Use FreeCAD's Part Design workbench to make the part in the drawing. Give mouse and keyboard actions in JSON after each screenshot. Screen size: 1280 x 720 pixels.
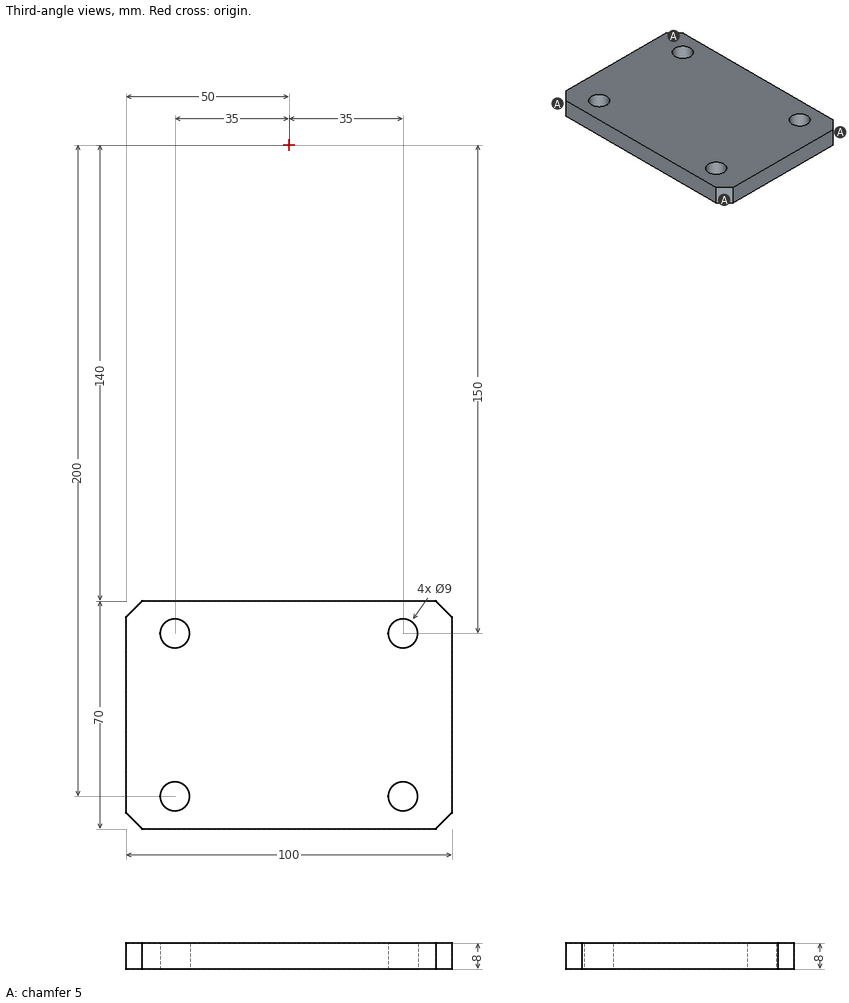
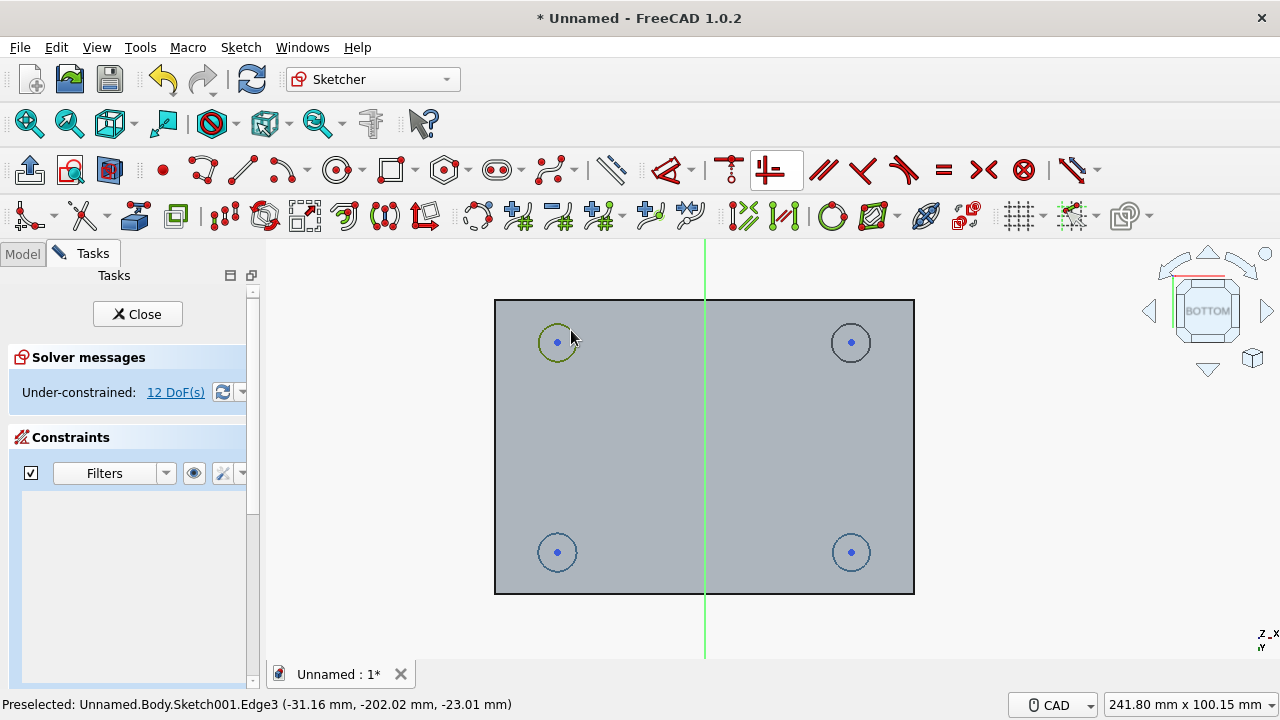
{"action": "left_click", "coordinate": [864, 329]}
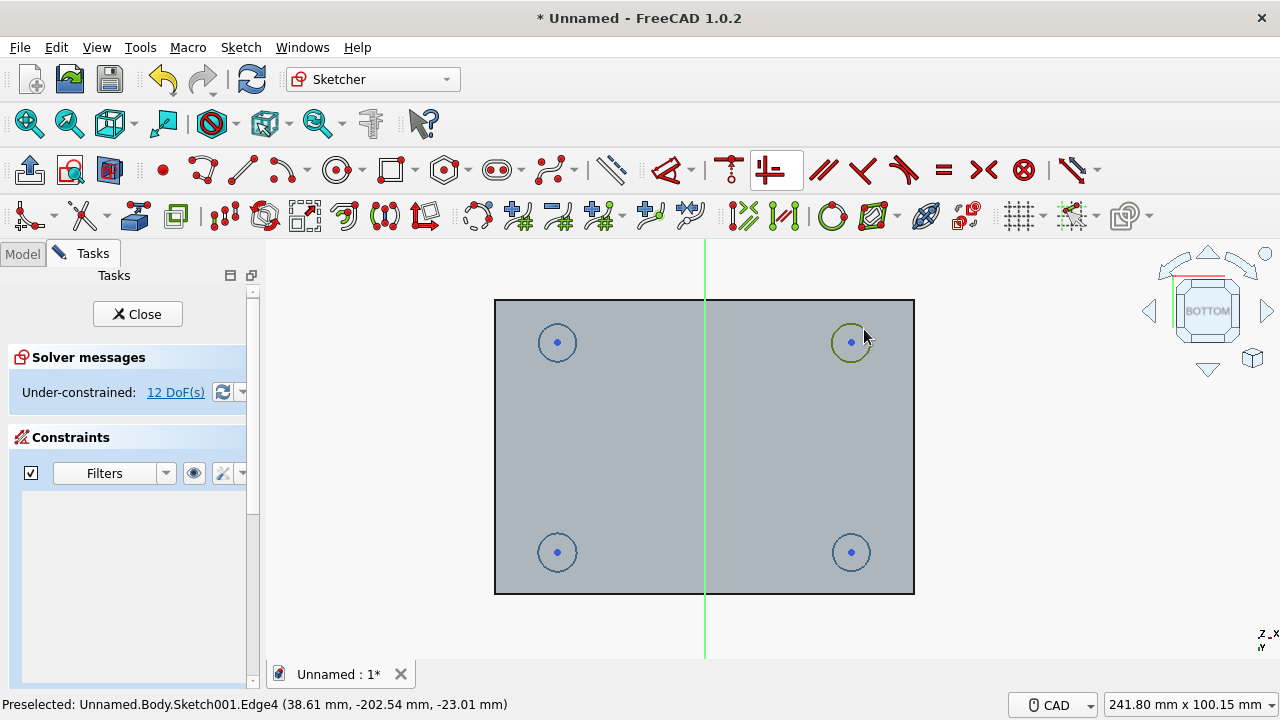
{"action": "left_click", "coordinate": [944, 170]}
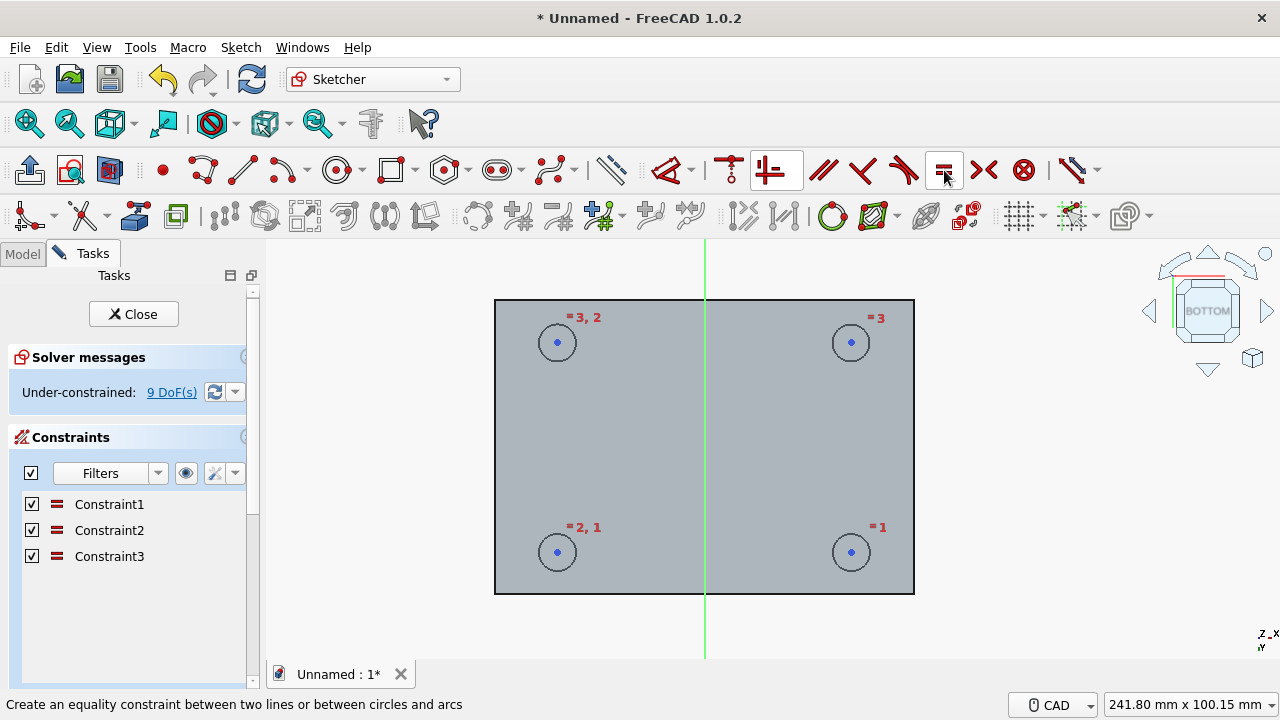
{"action": "left_click", "coordinate": [851, 553]}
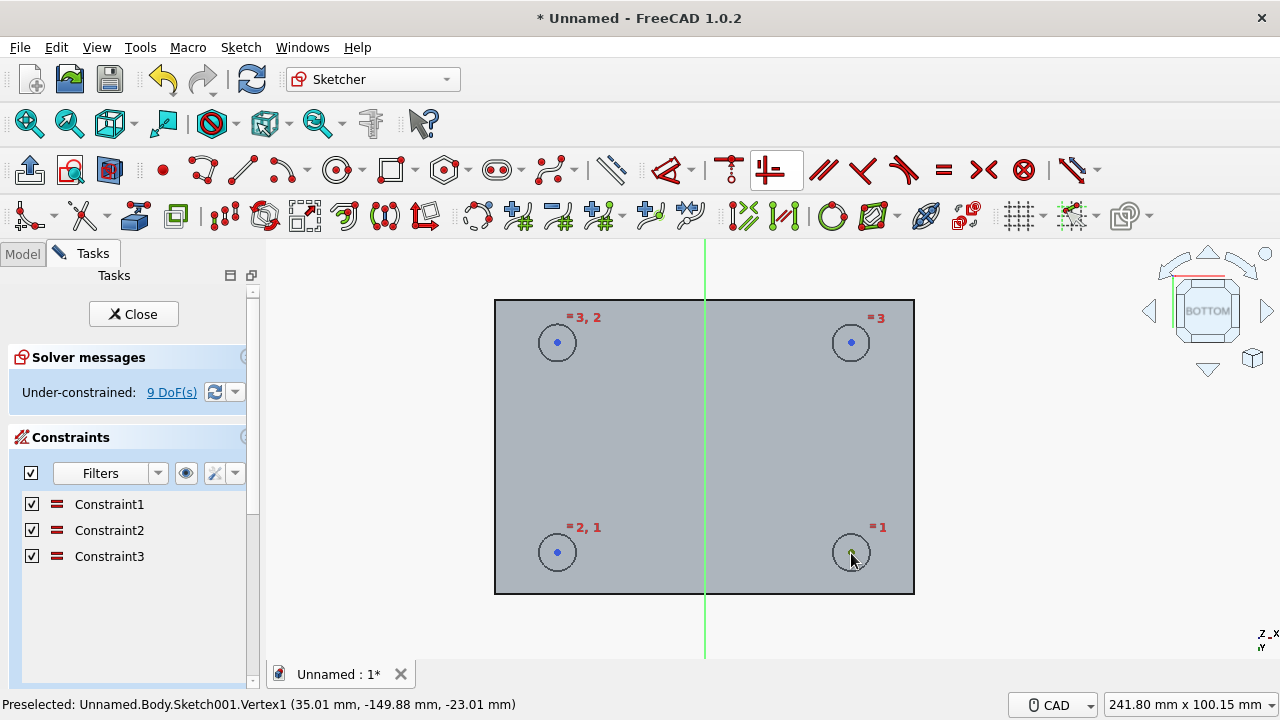
{"action": "left_click", "coordinate": [557, 553]}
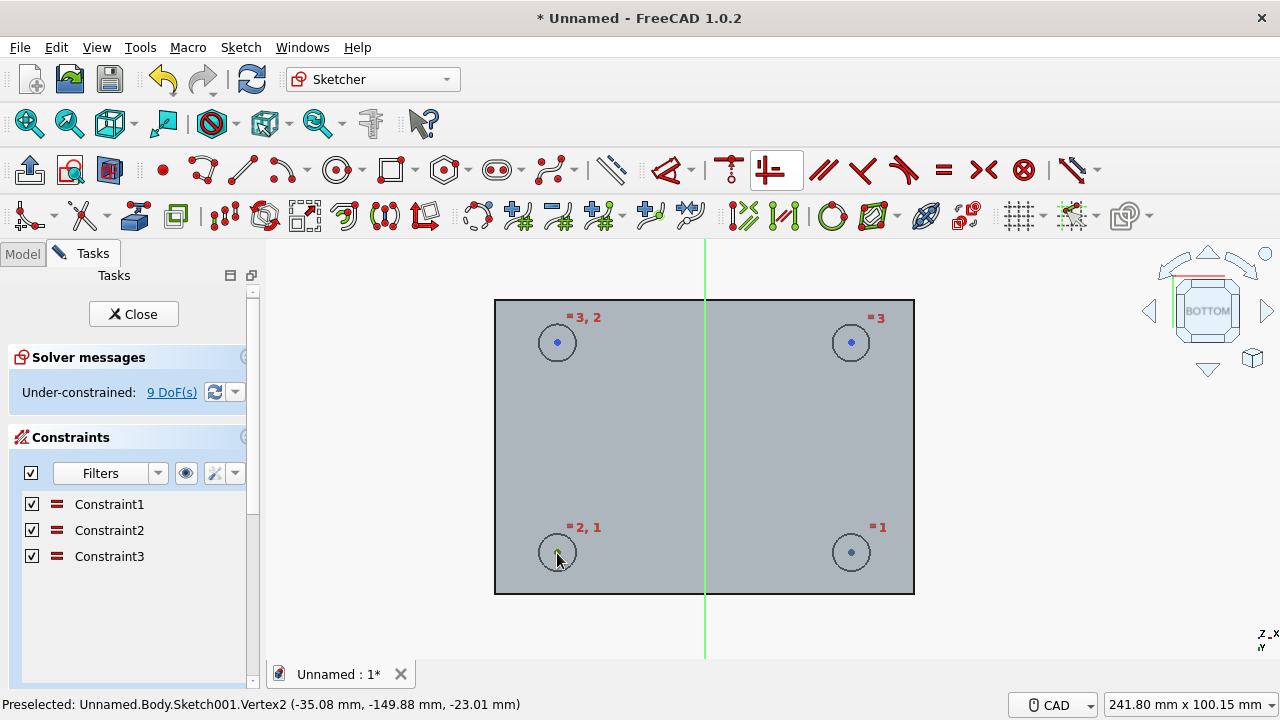
{"action": "left_click", "coordinate": [798, 170]}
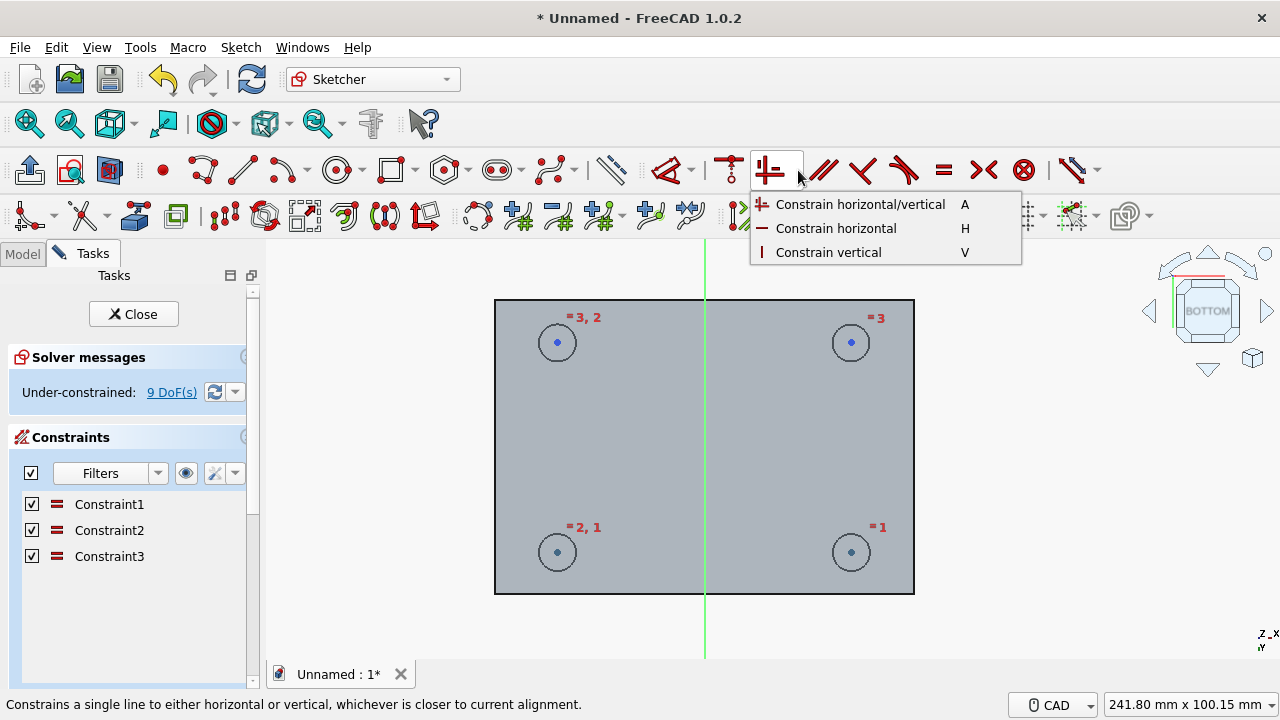
{"action": "left_click", "coordinate": [886, 228]}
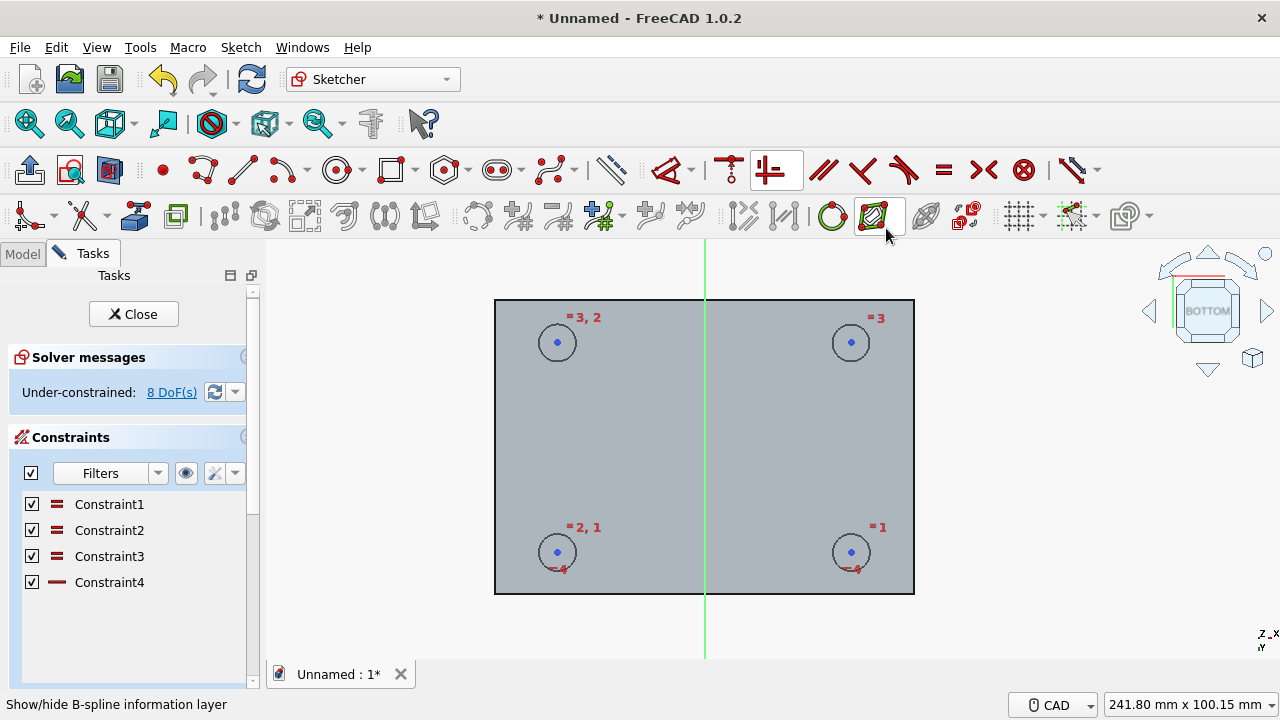
{"action": "left_click", "coordinate": [557, 553]}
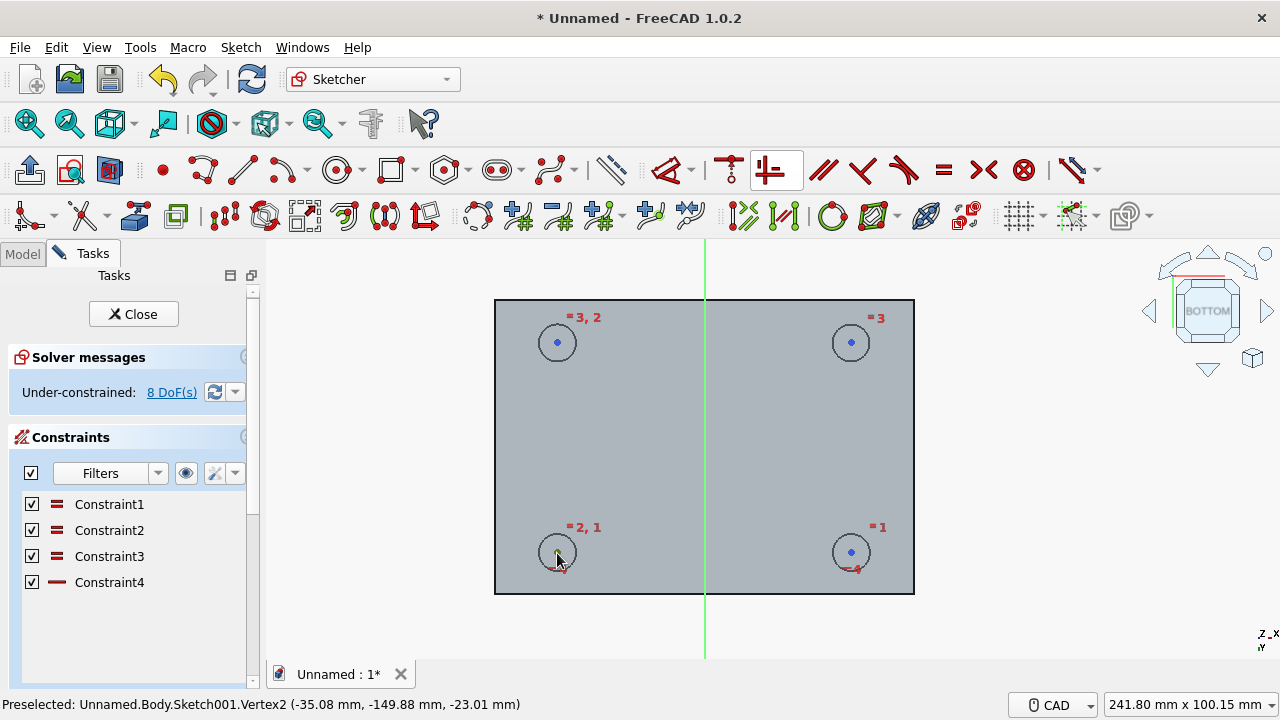
{"action": "left_click", "coordinate": [557, 343]}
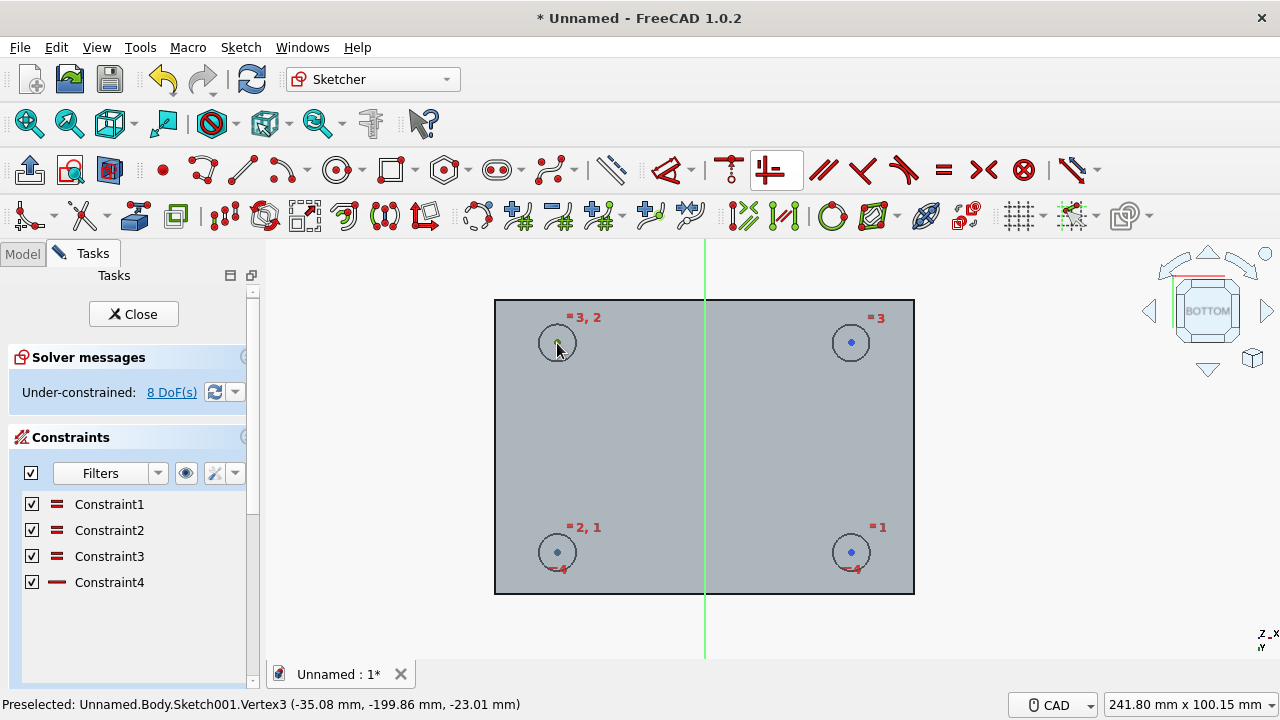
{"action": "left_click", "coordinate": [798, 170]}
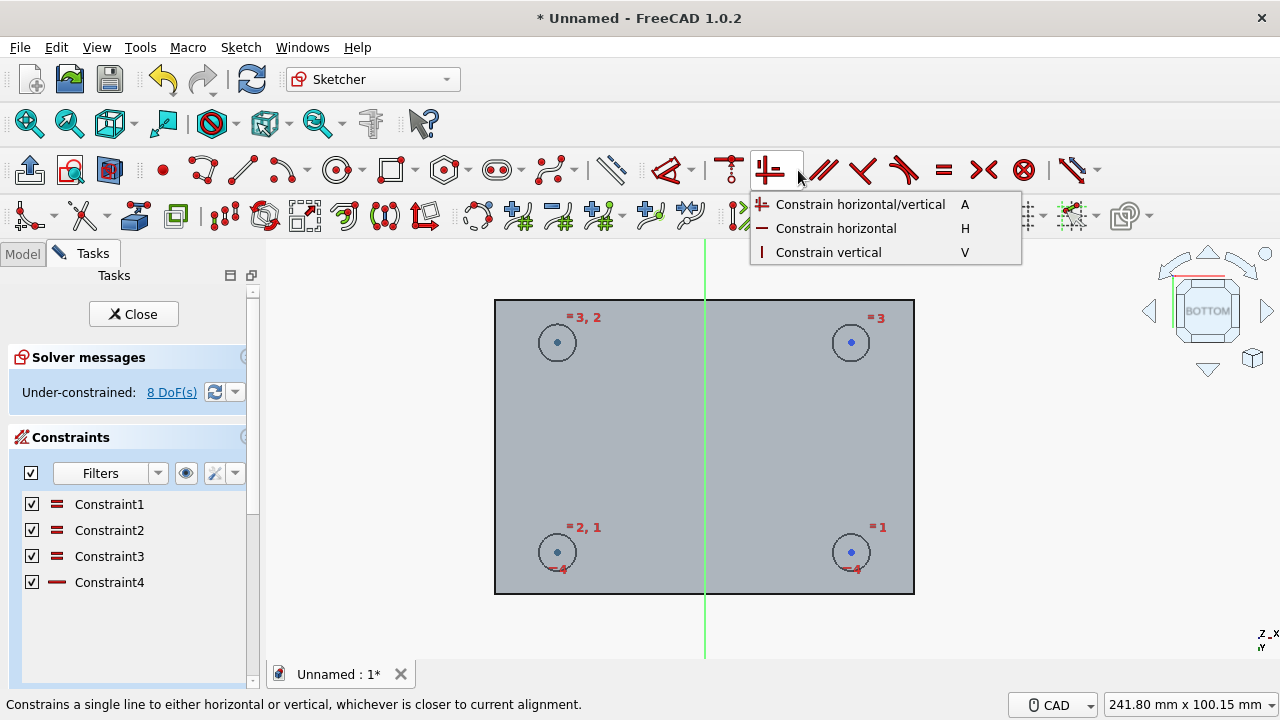
{"action": "left_click", "coordinate": [886, 252]}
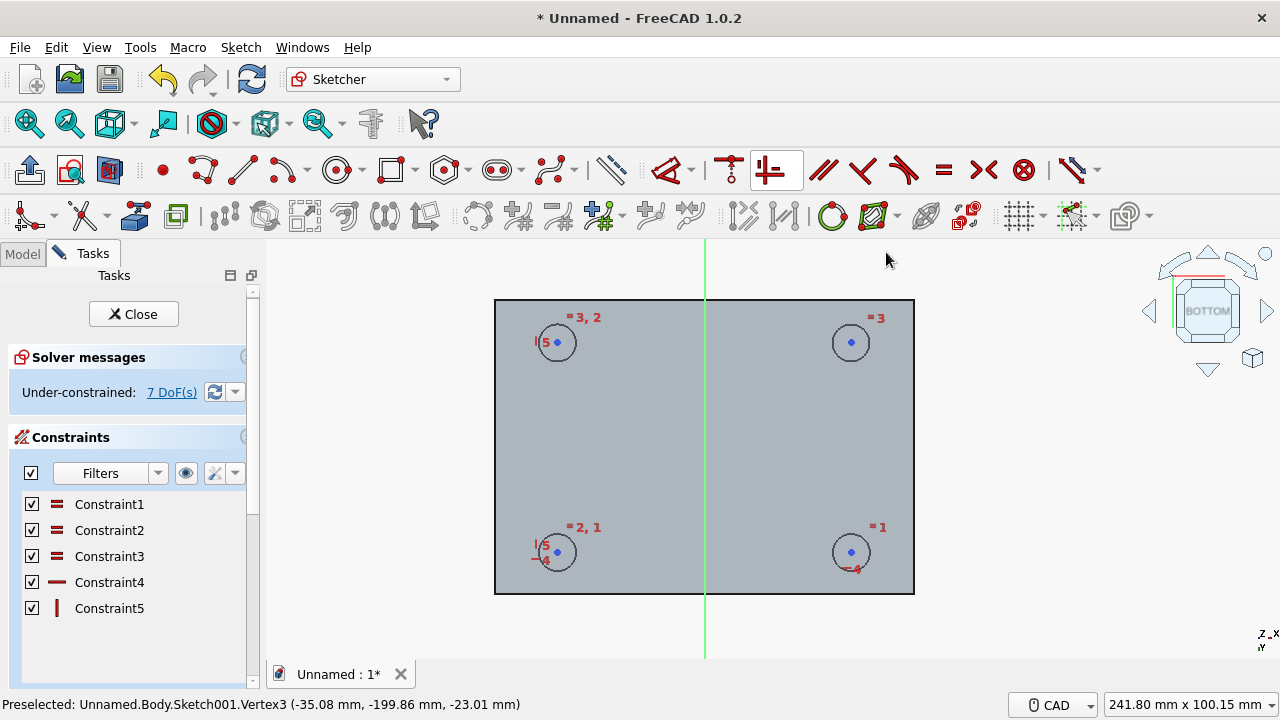
{"action": "left_click", "coordinate": [851, 553]}